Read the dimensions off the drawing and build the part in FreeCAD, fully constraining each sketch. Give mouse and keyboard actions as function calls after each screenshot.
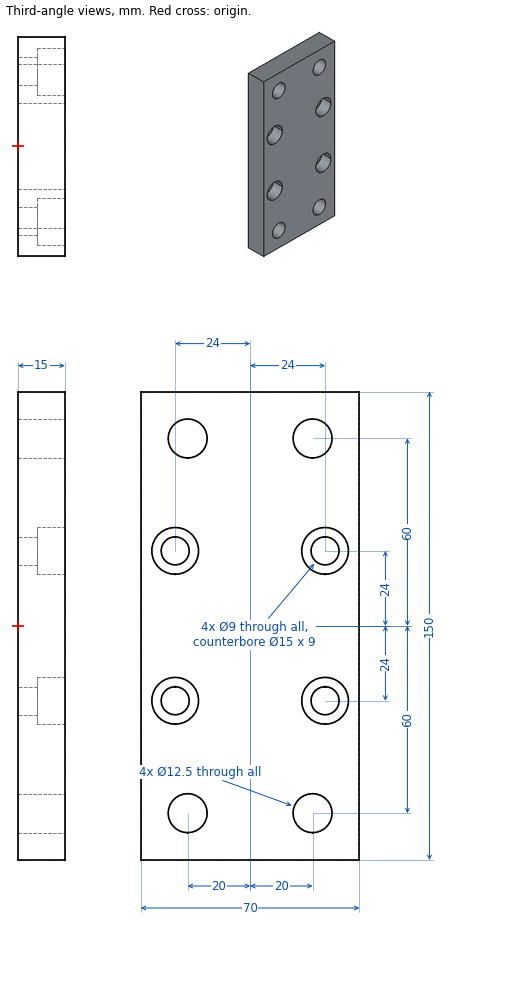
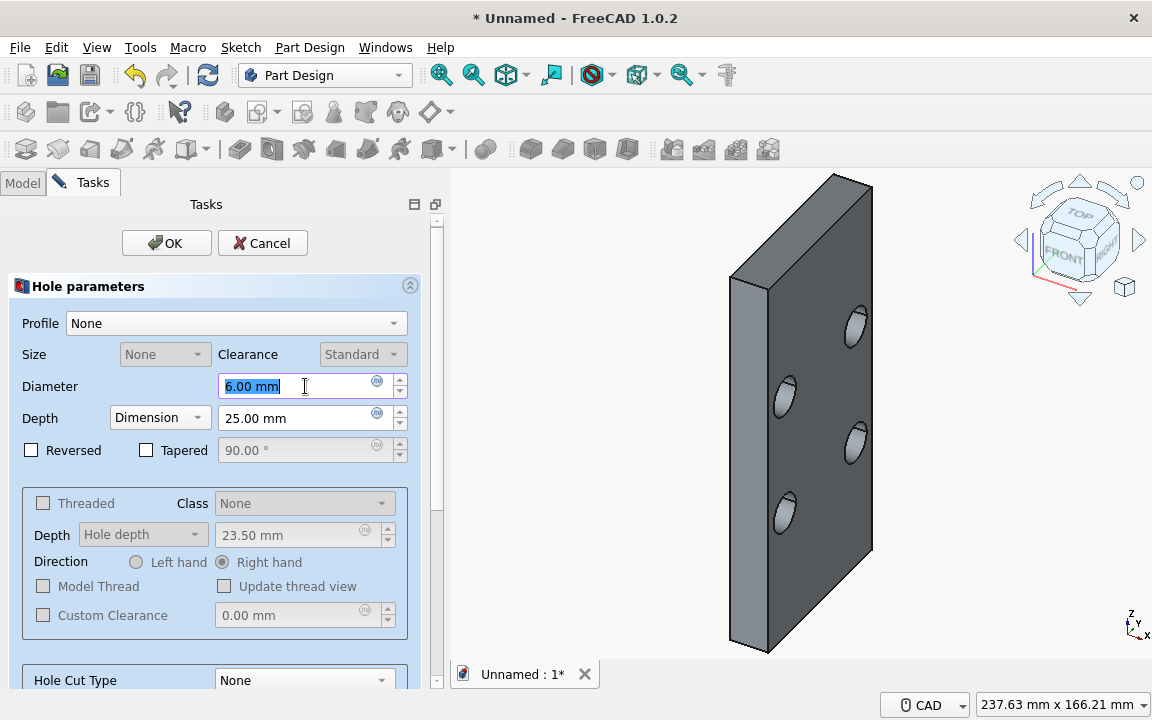
text(12.5)
key(Tab)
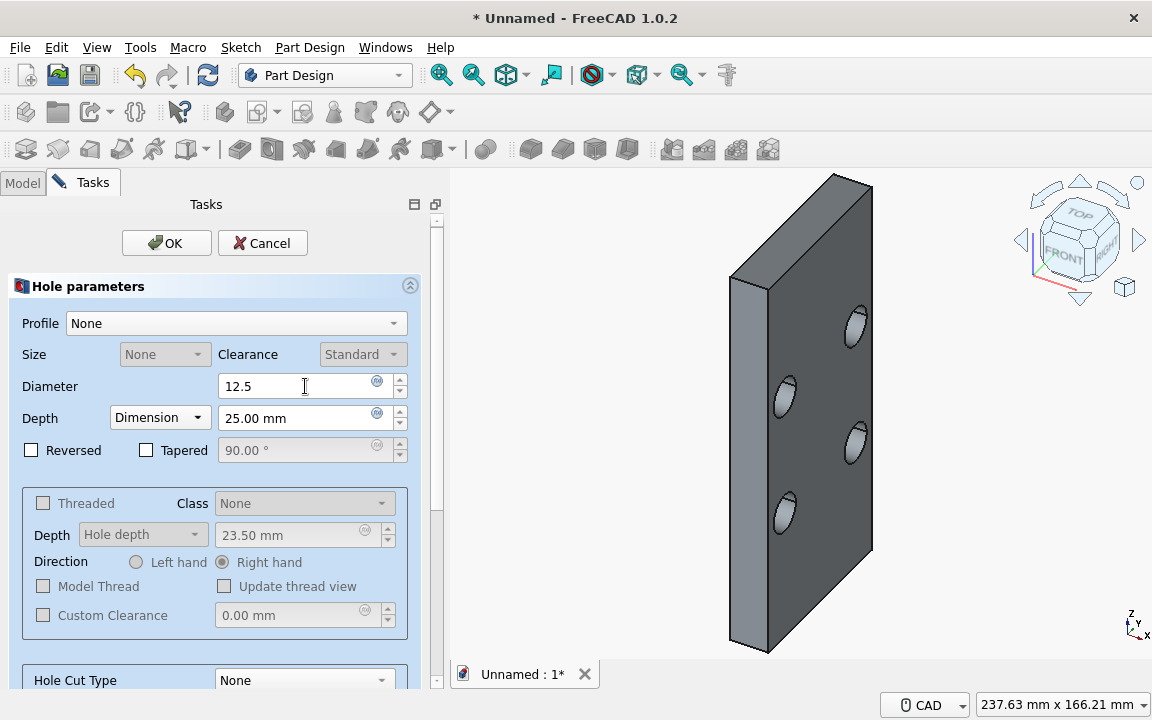
click(161, 418)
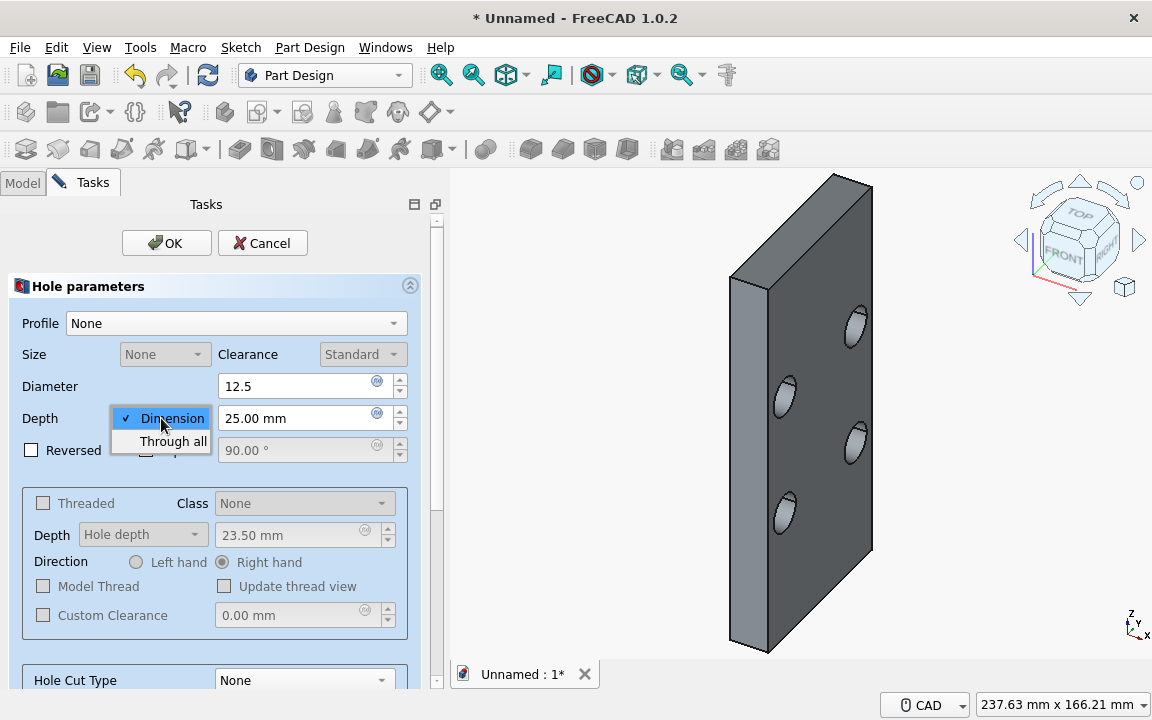
click(160, 442)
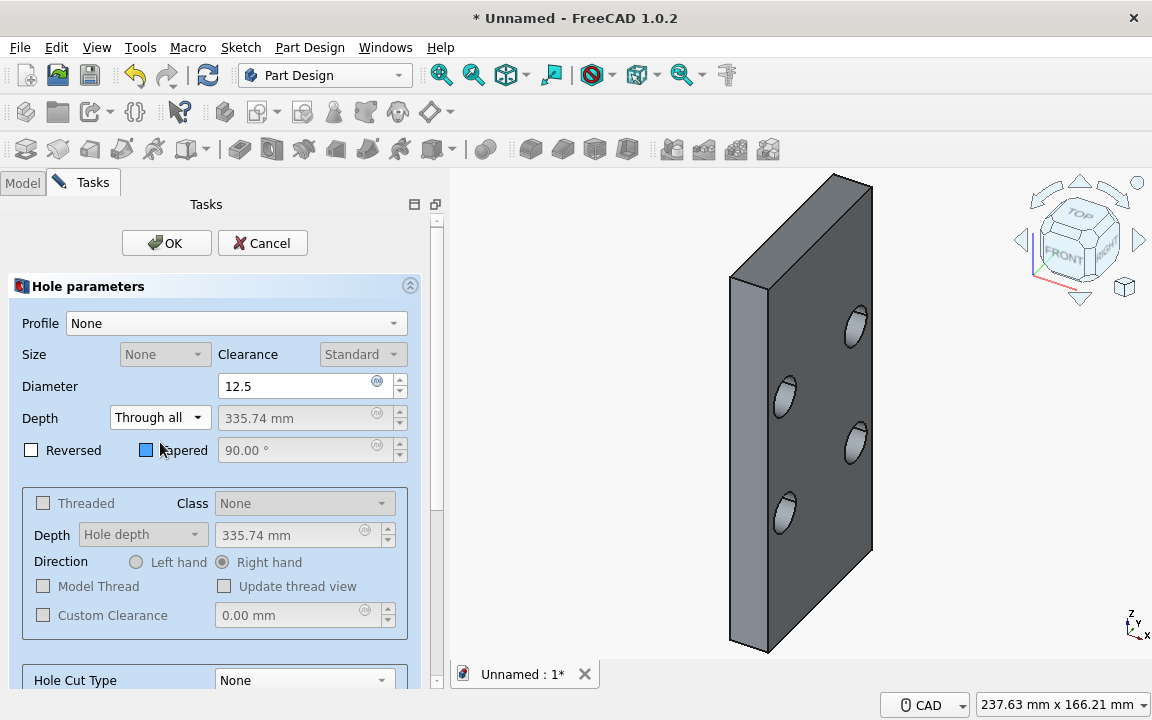
click(30, 450)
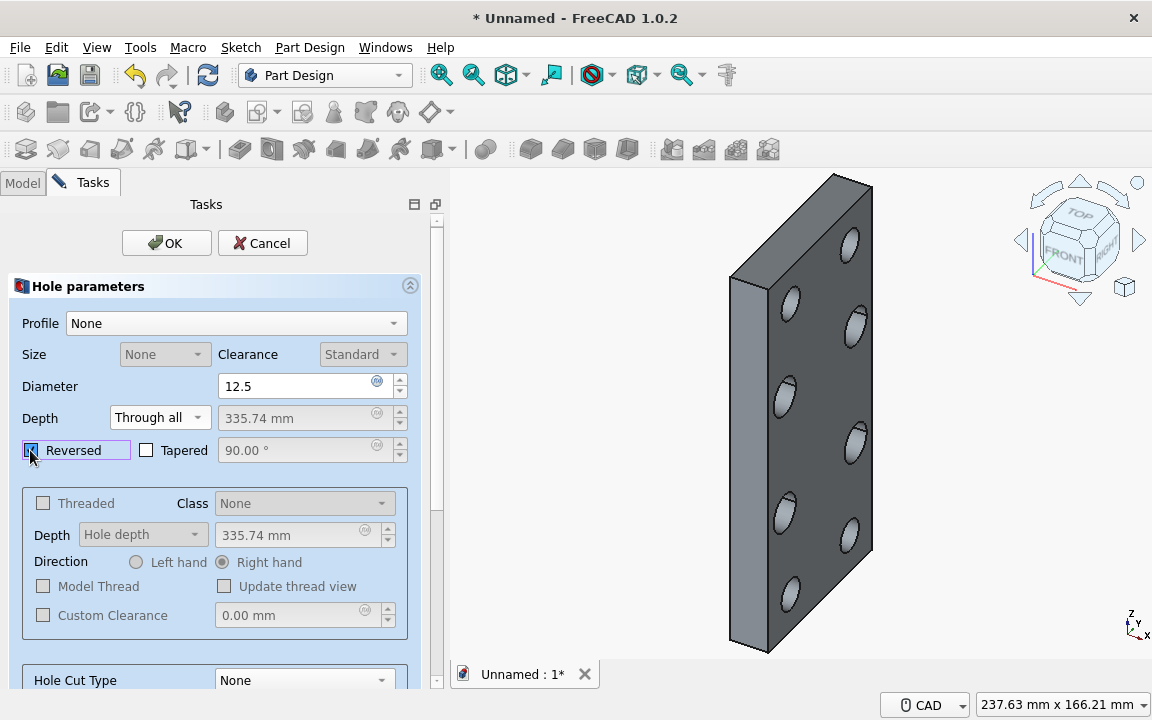
click(167, 243)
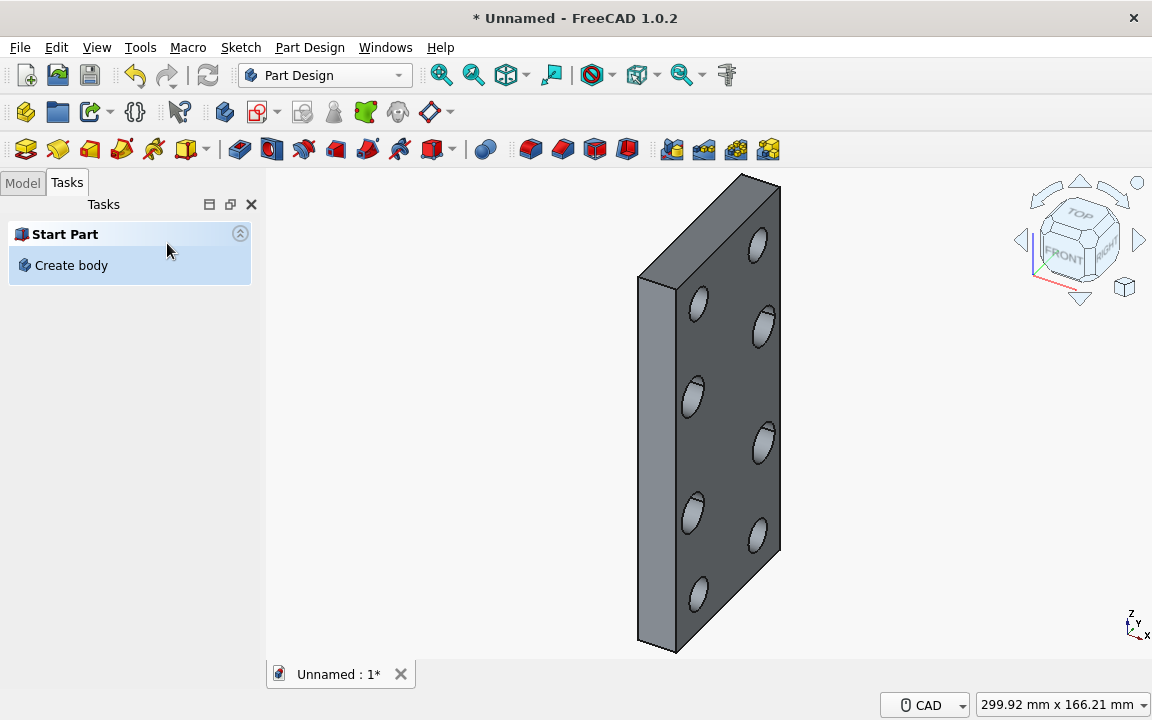
key(0)